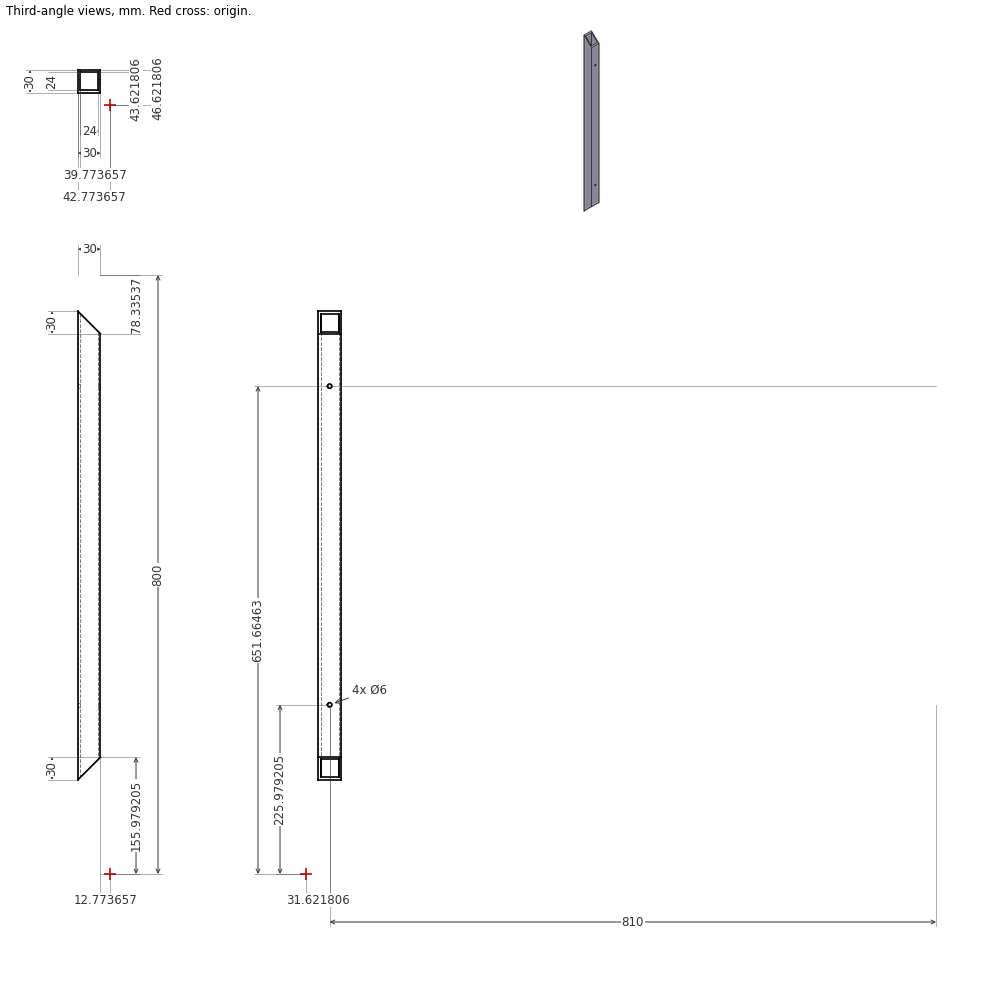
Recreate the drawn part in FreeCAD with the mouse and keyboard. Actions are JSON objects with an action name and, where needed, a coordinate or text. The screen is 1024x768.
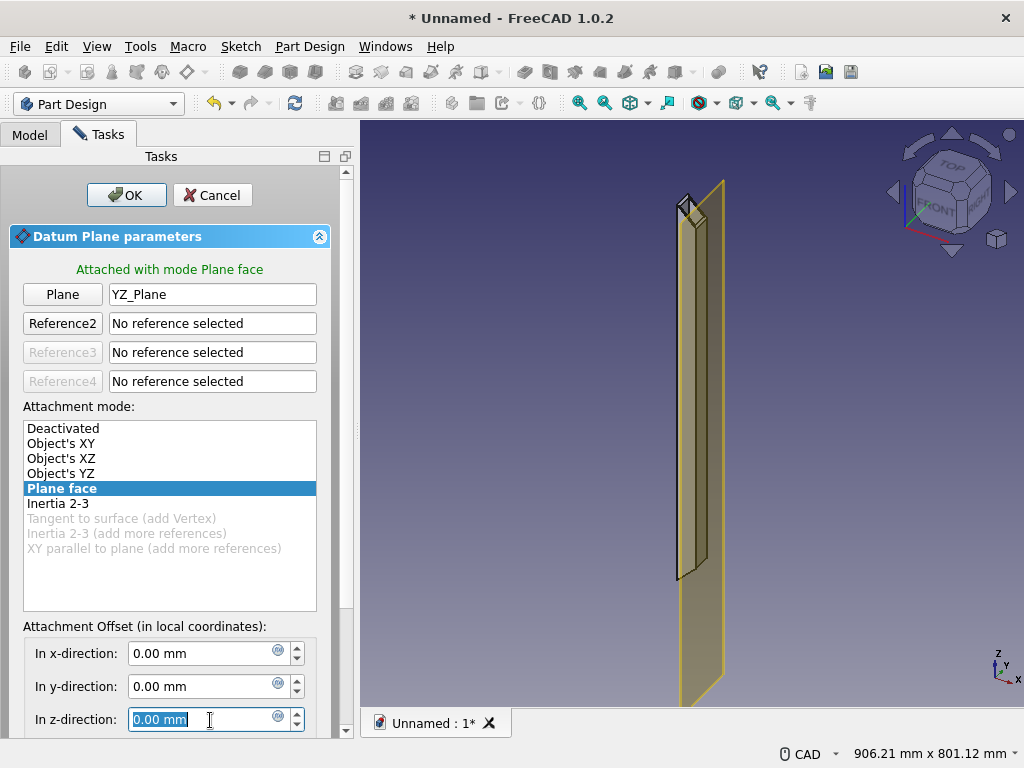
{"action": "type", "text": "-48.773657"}
{"action": "key", "text": "Tab"}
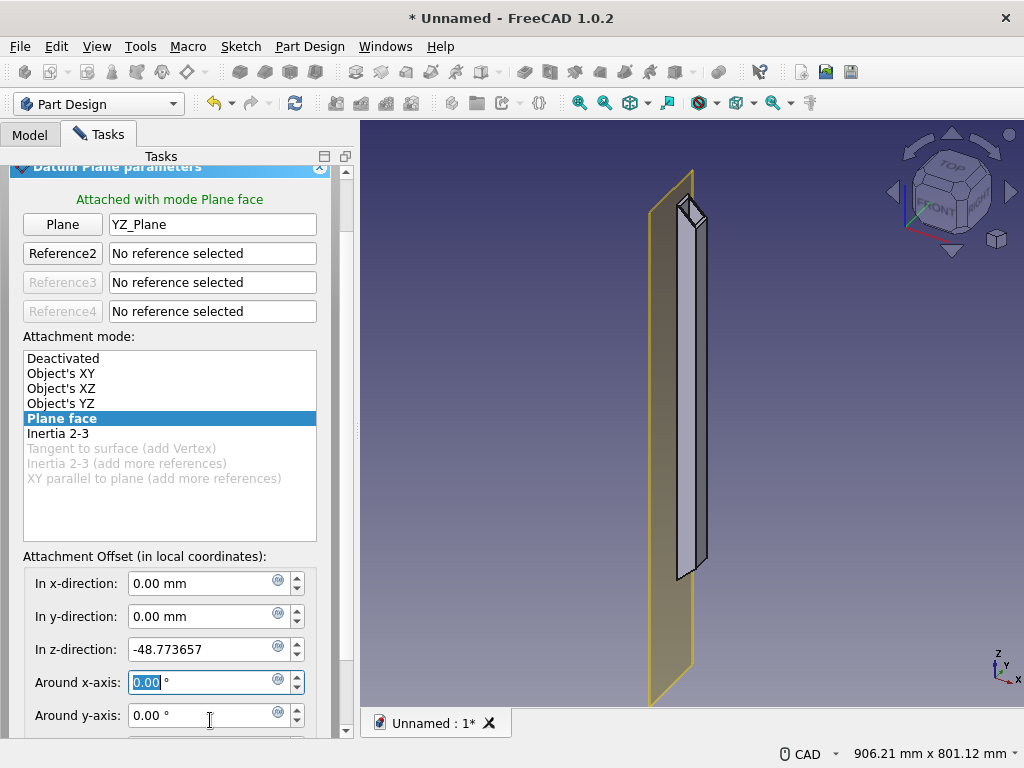
{"action": "scroll", "coordinate": [346, 452], "scroll_direction": "up", "scroll_amount": 2}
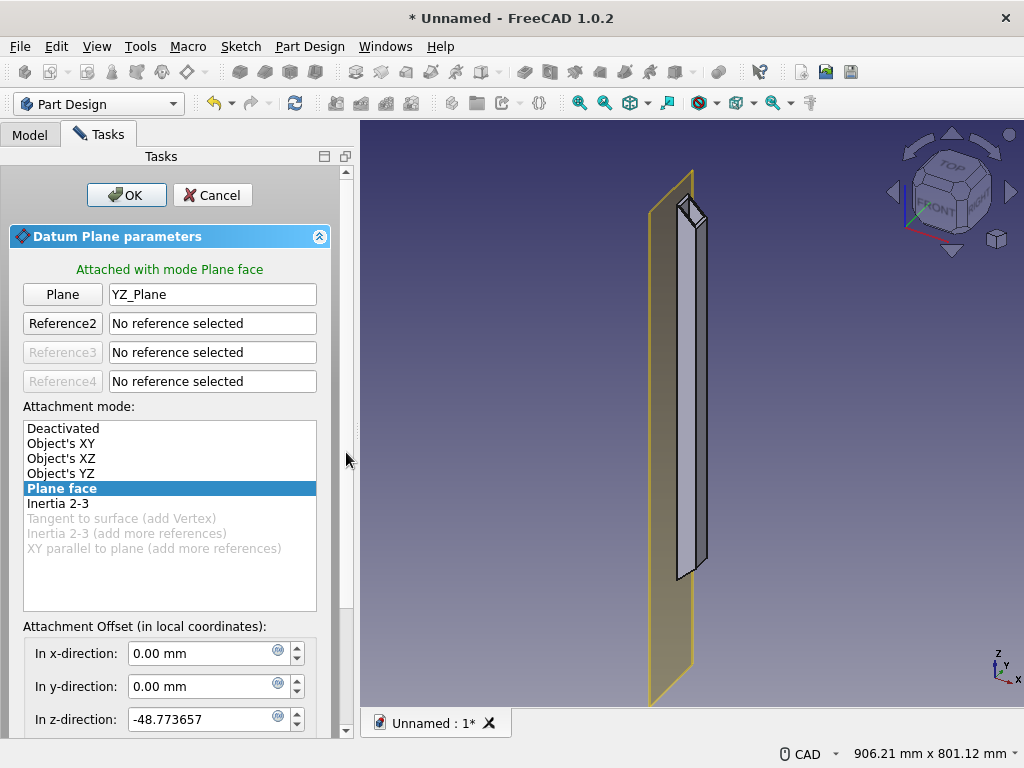
{"action": "left_click", "coordinate": [127, 195]}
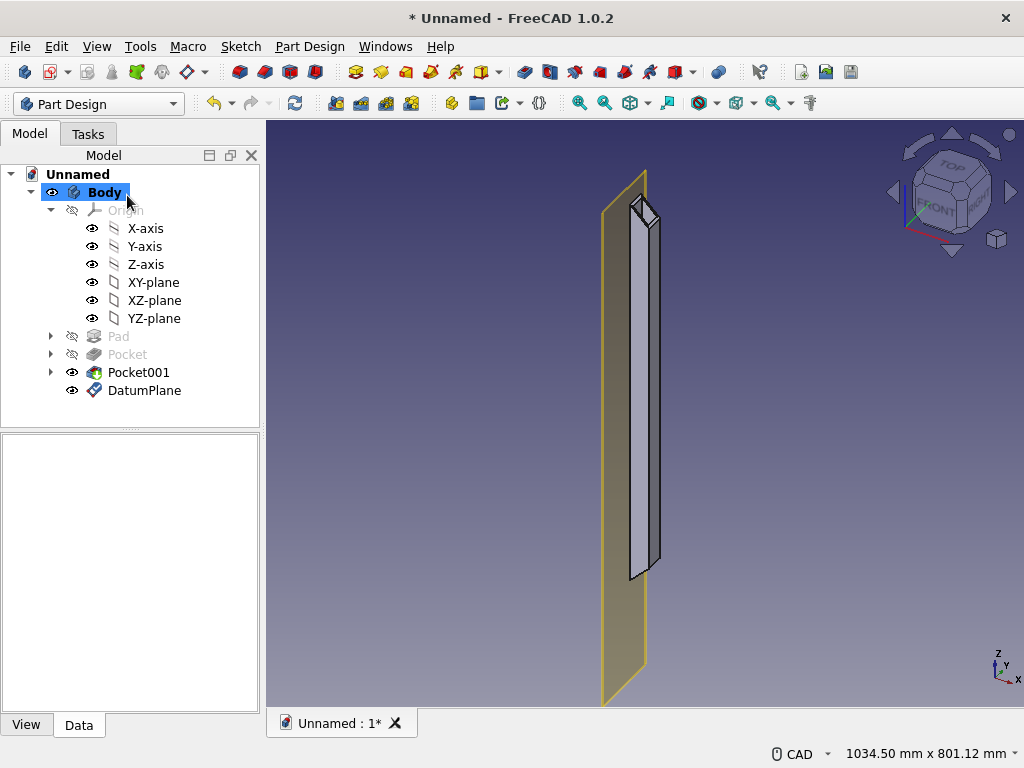
{"action": "left_click", "coordinate": [117, 390]}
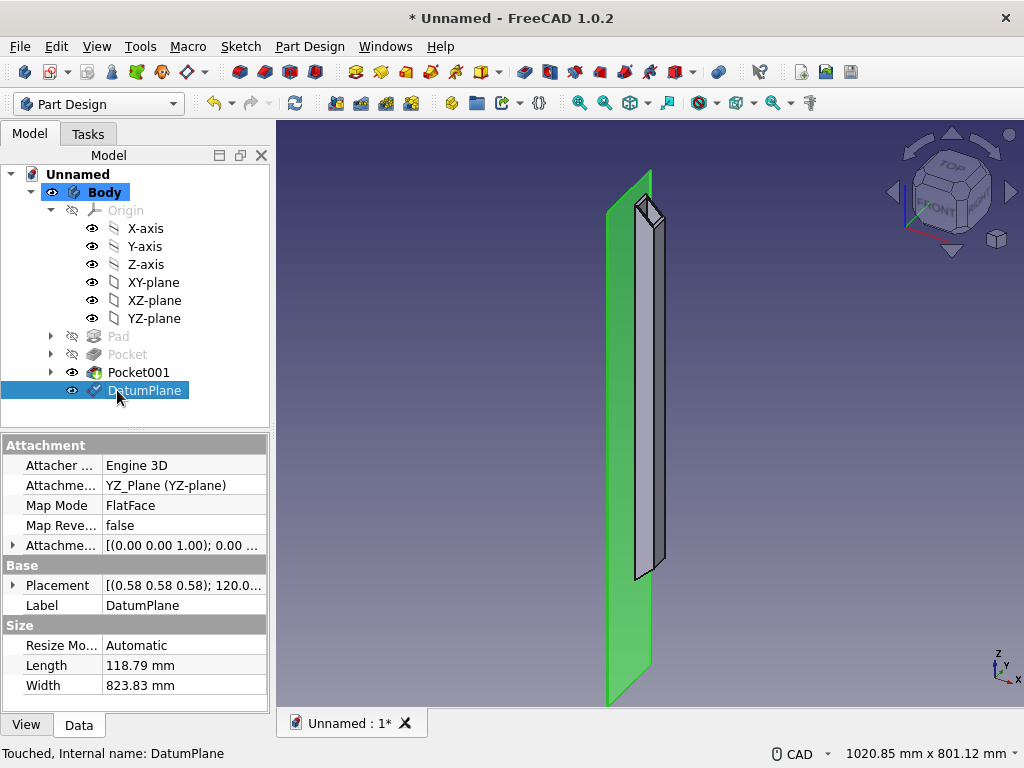
{"action": "left_click", "coordinate": [50, 72]}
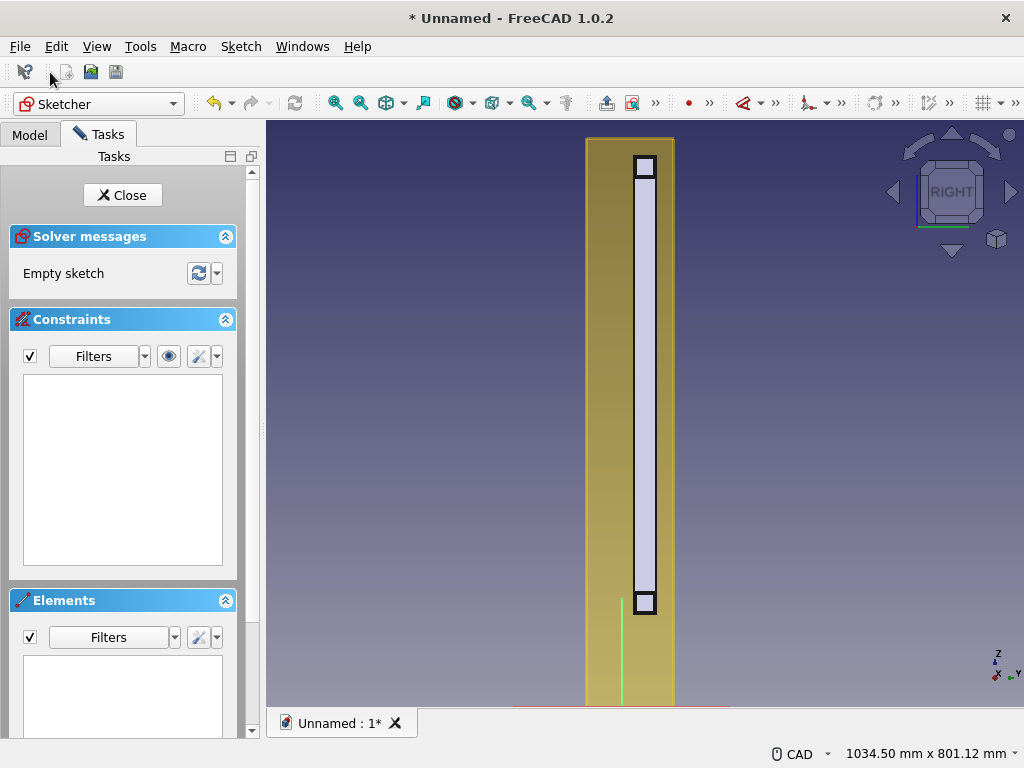
{"action": "key", "text": "q s"}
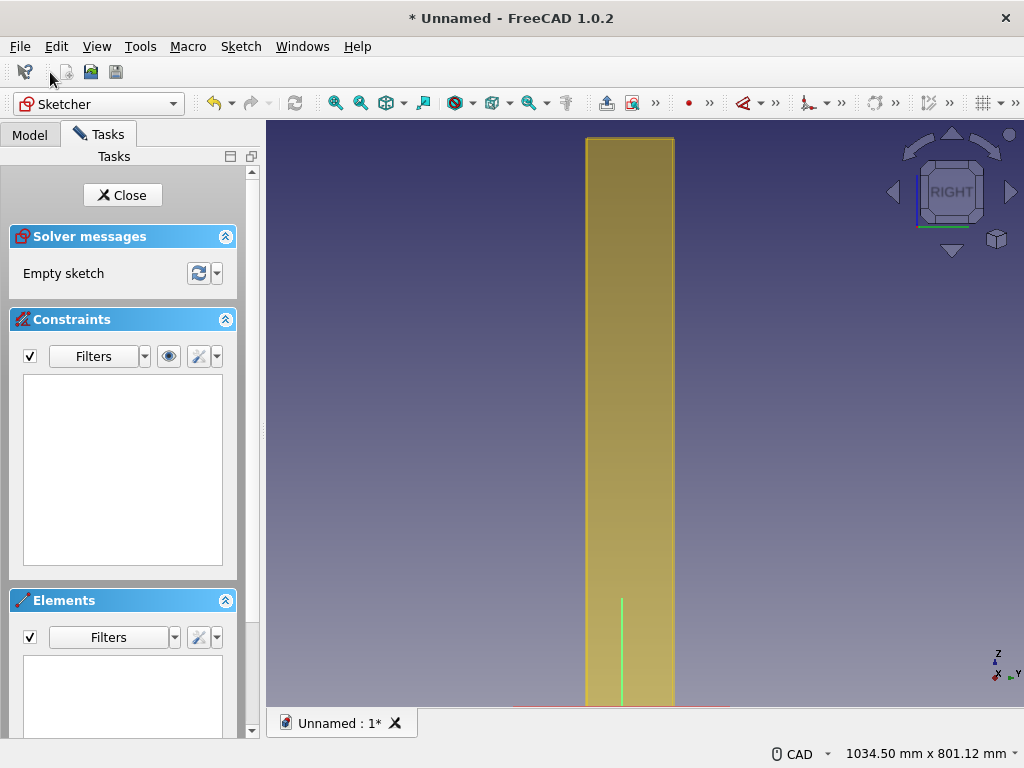
{"action": "scroll", "coordinate": [294, 349], "scroll_direction": "down", "scroll_amount": 3}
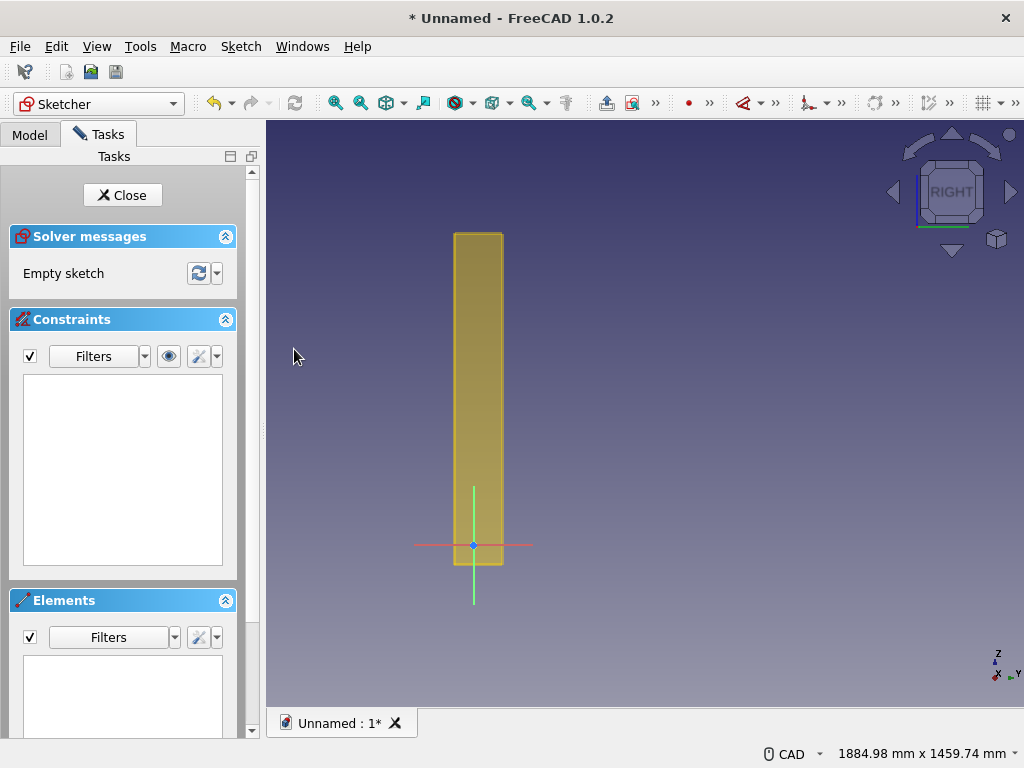
{"action": "key", "text": "g c"}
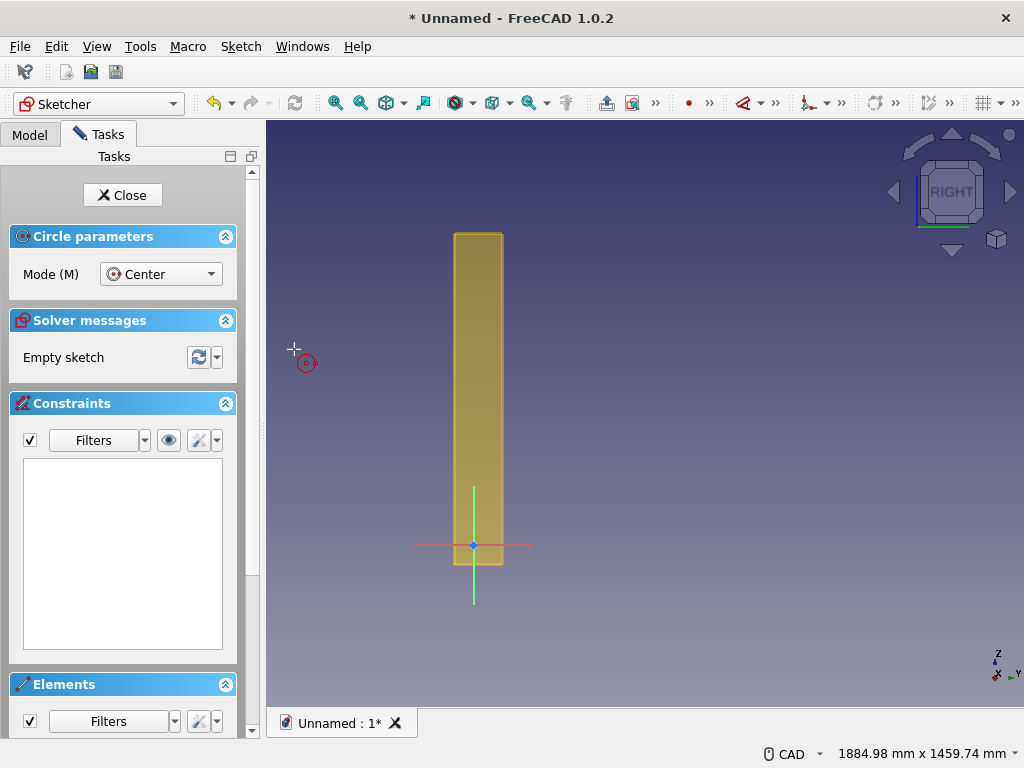
{"action": "scroll", "coordinate": [487, 455], "scroll_direction": "up", "scroll_amount": 15}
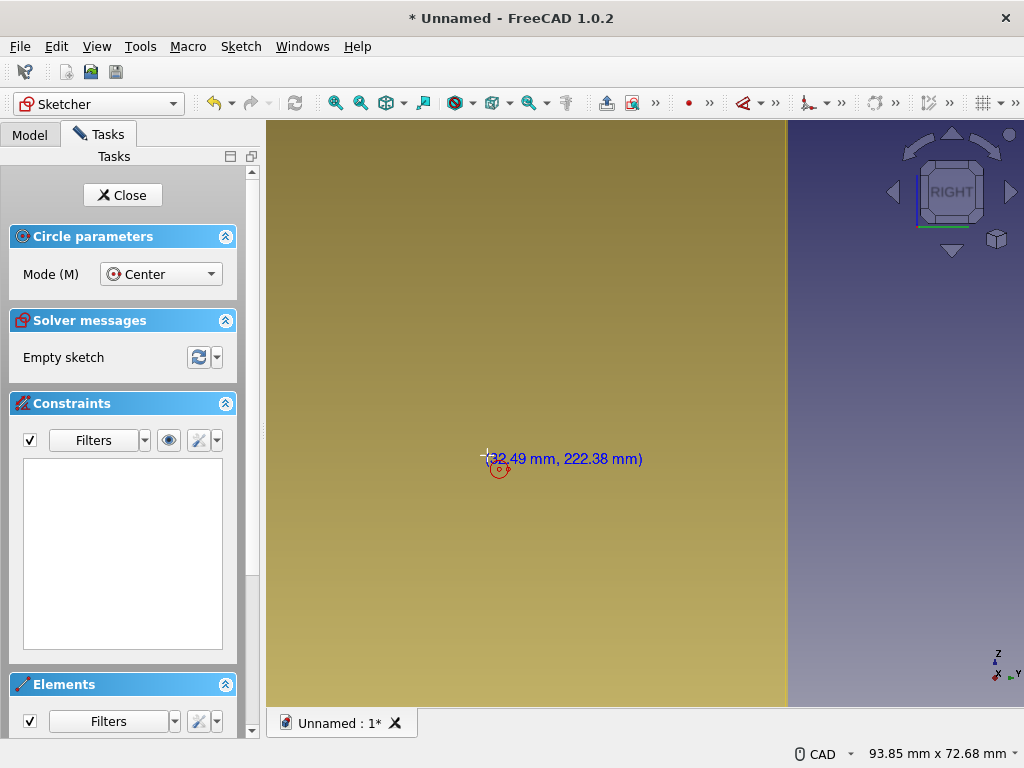
{"action": "scroll", "coordinate": [379, 465], "scroll_direction": "down", "scroll_amount": 14}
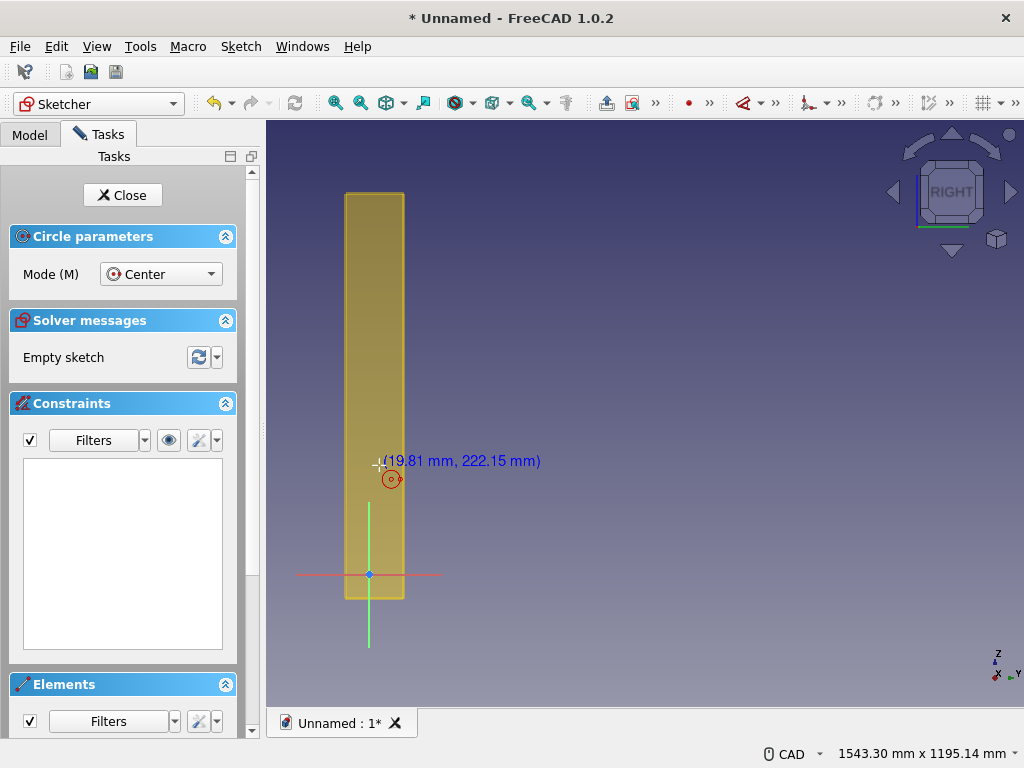
{"action": "left_click", "coordinate": [385, 464]}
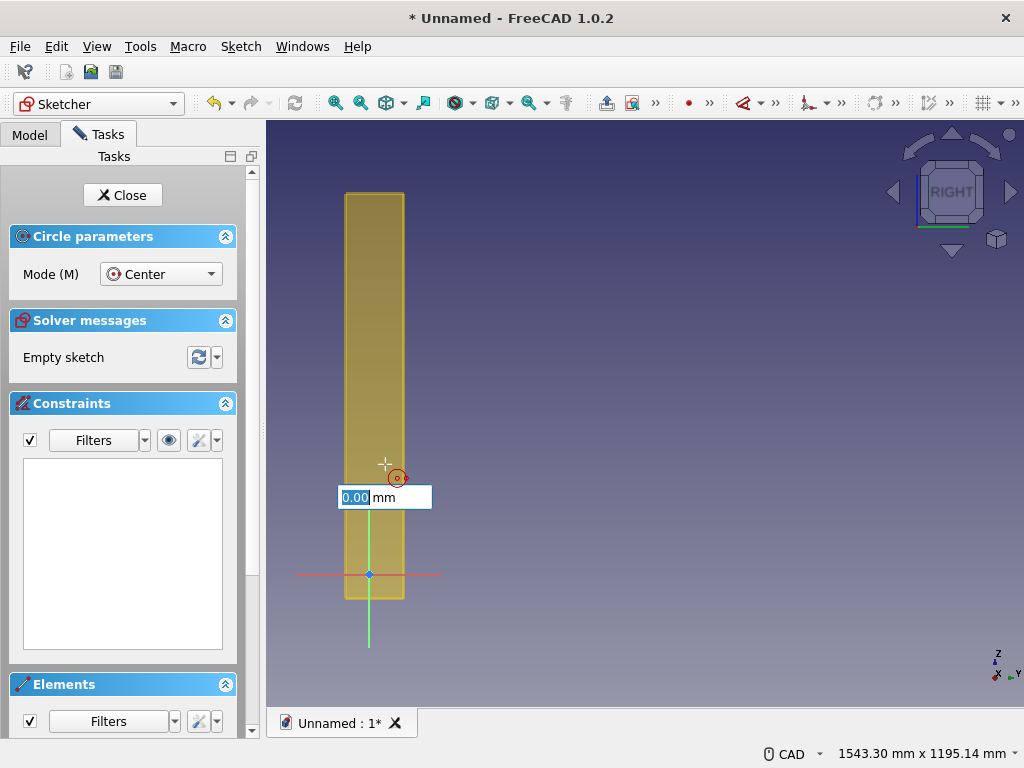
{"action": "scroll", "coordinate": [386, 463], "scroll_direction": "up", "scroll_amount": 12}